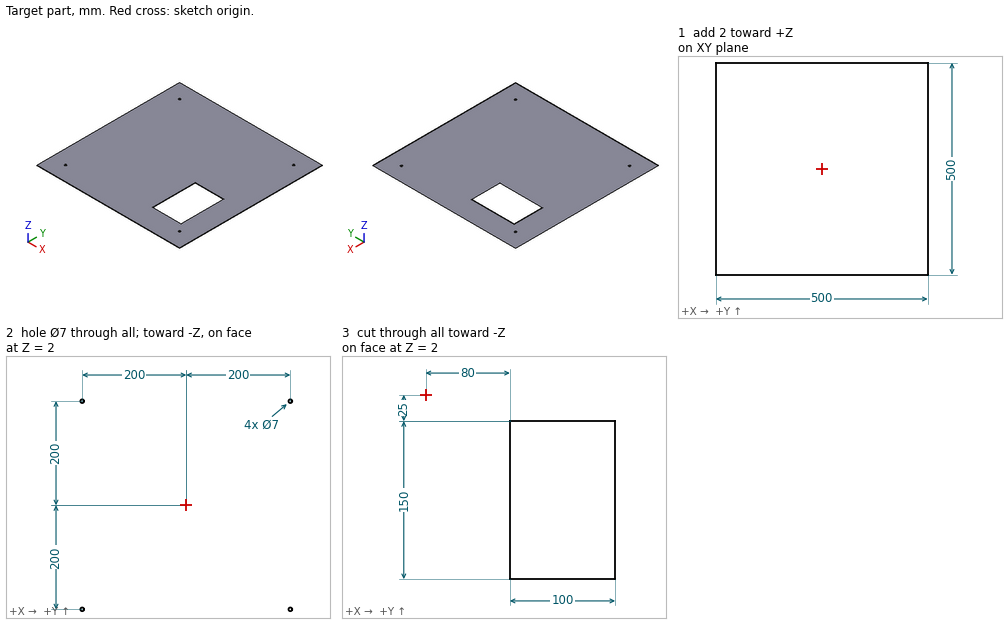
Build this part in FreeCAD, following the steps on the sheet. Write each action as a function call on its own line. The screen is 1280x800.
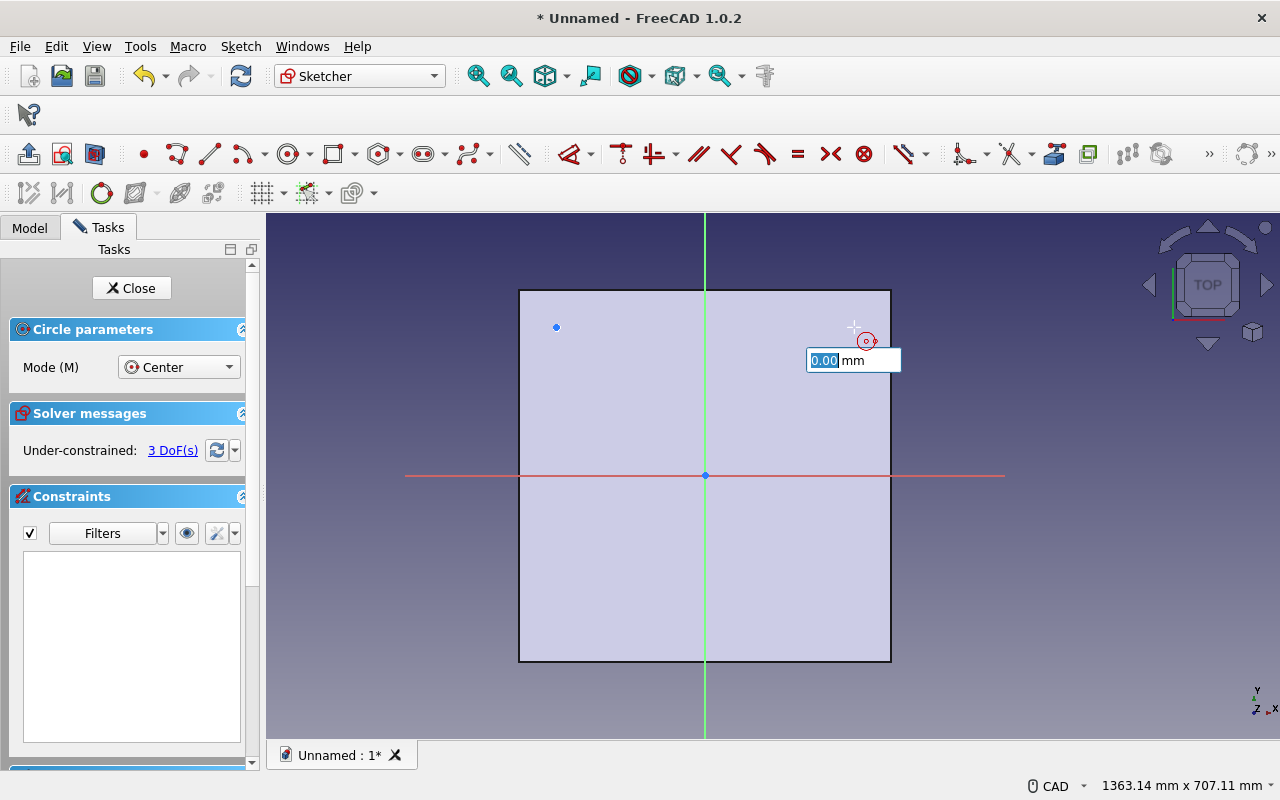
scroll(856, 325, up, 10)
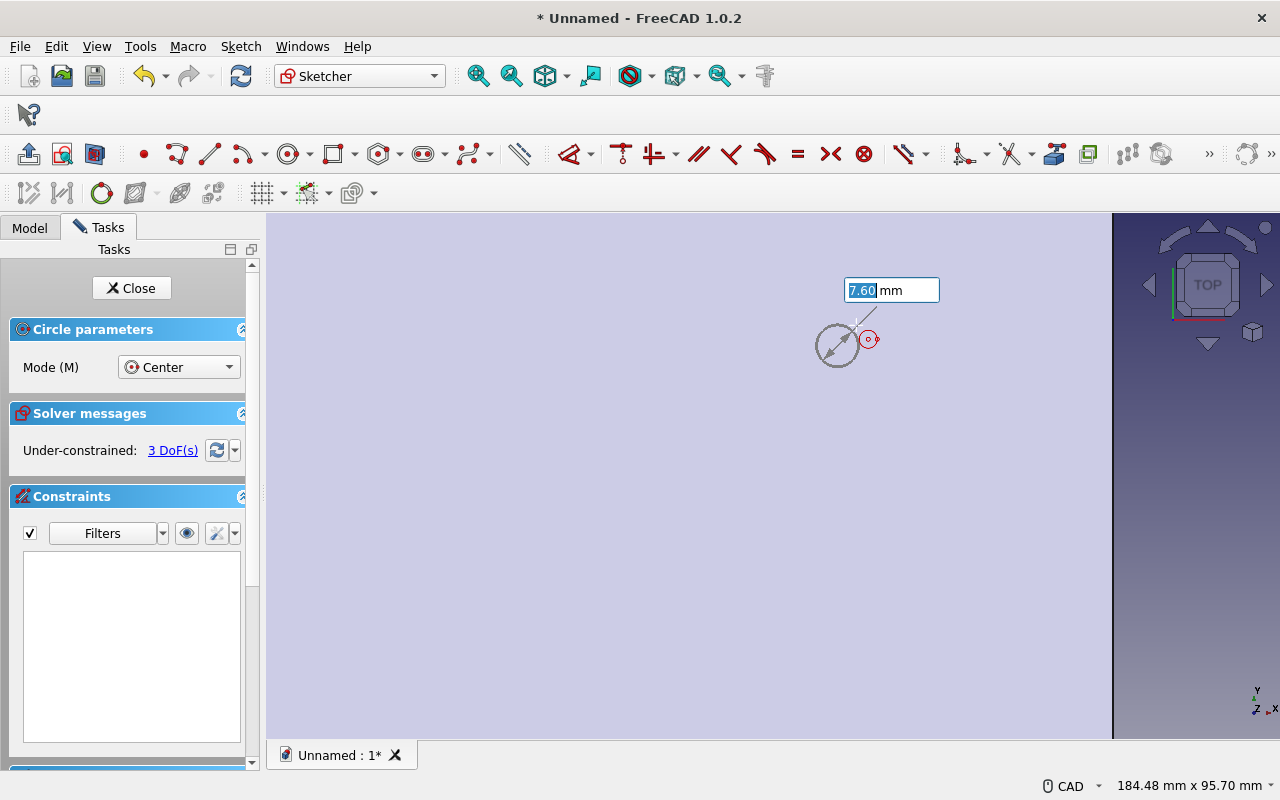
click(852, 326)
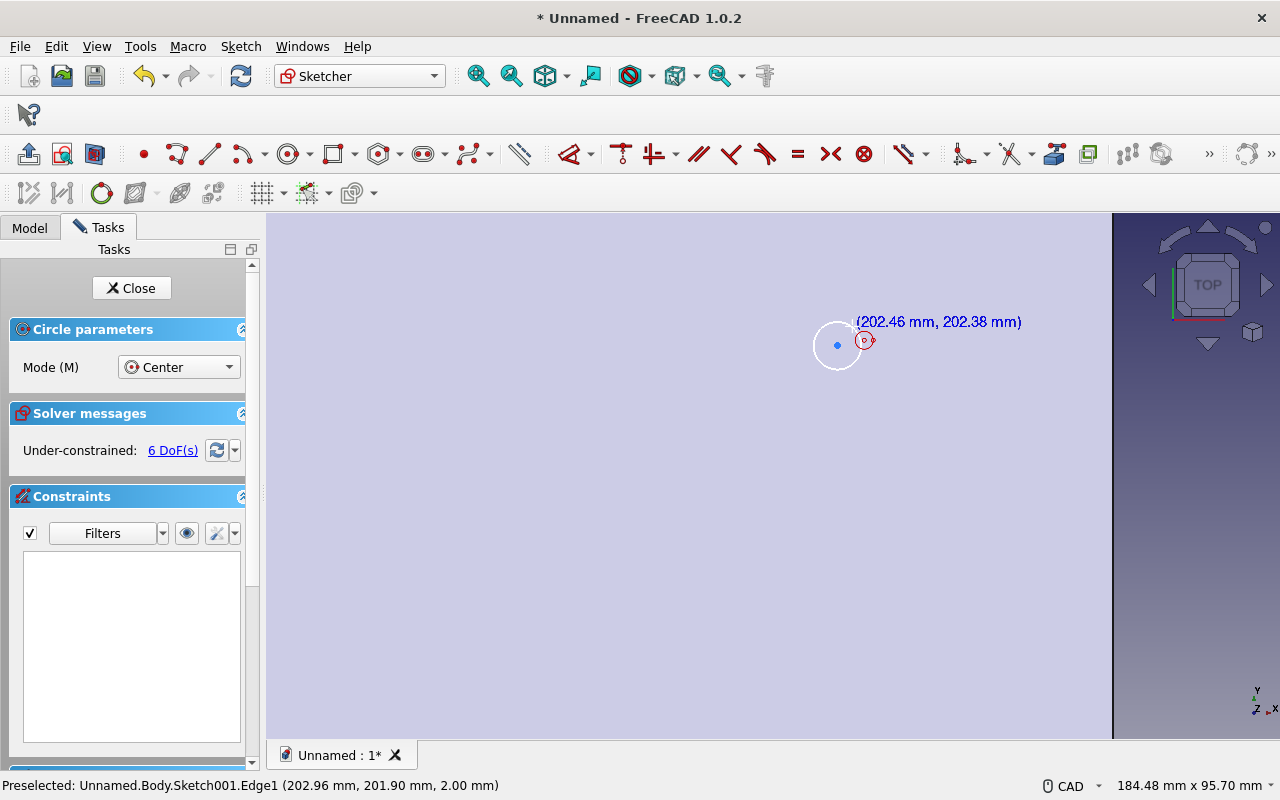
scroll(856, 325, down, 10)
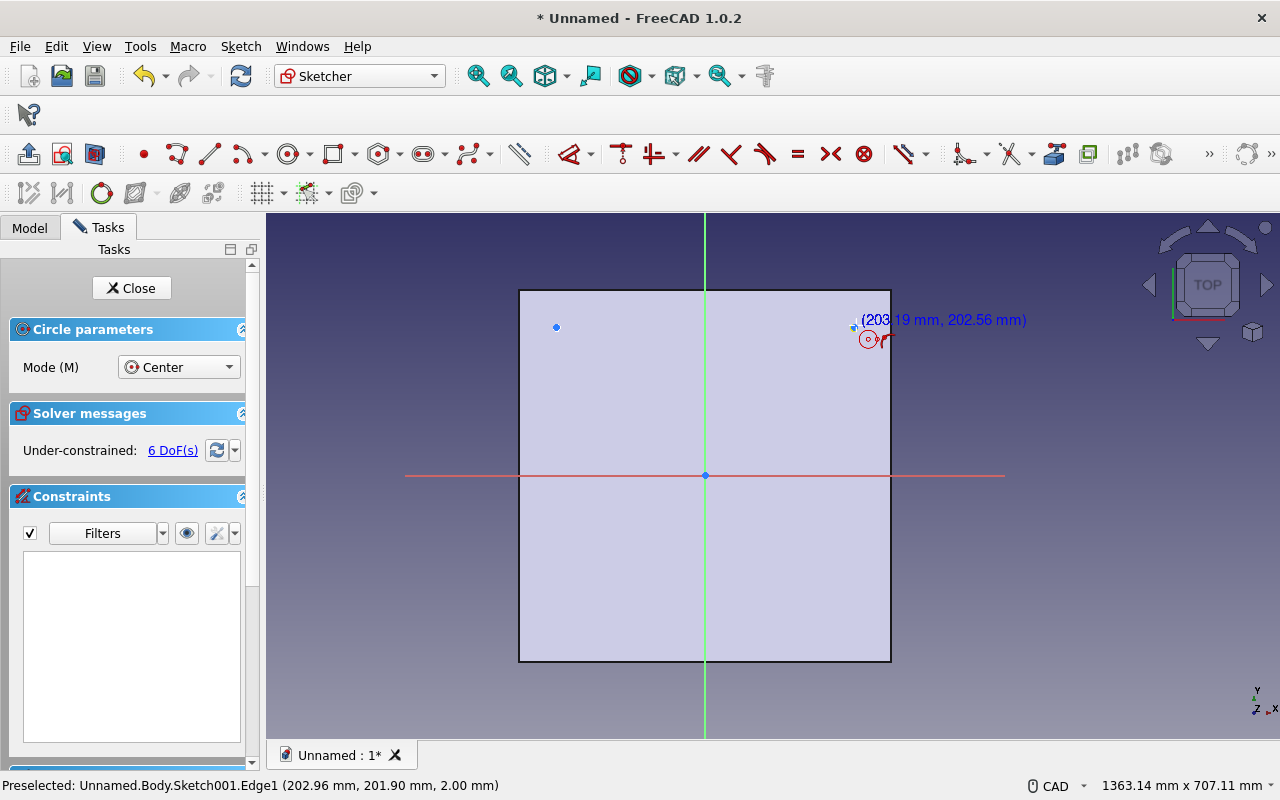
scroll(557, 625, up, 11)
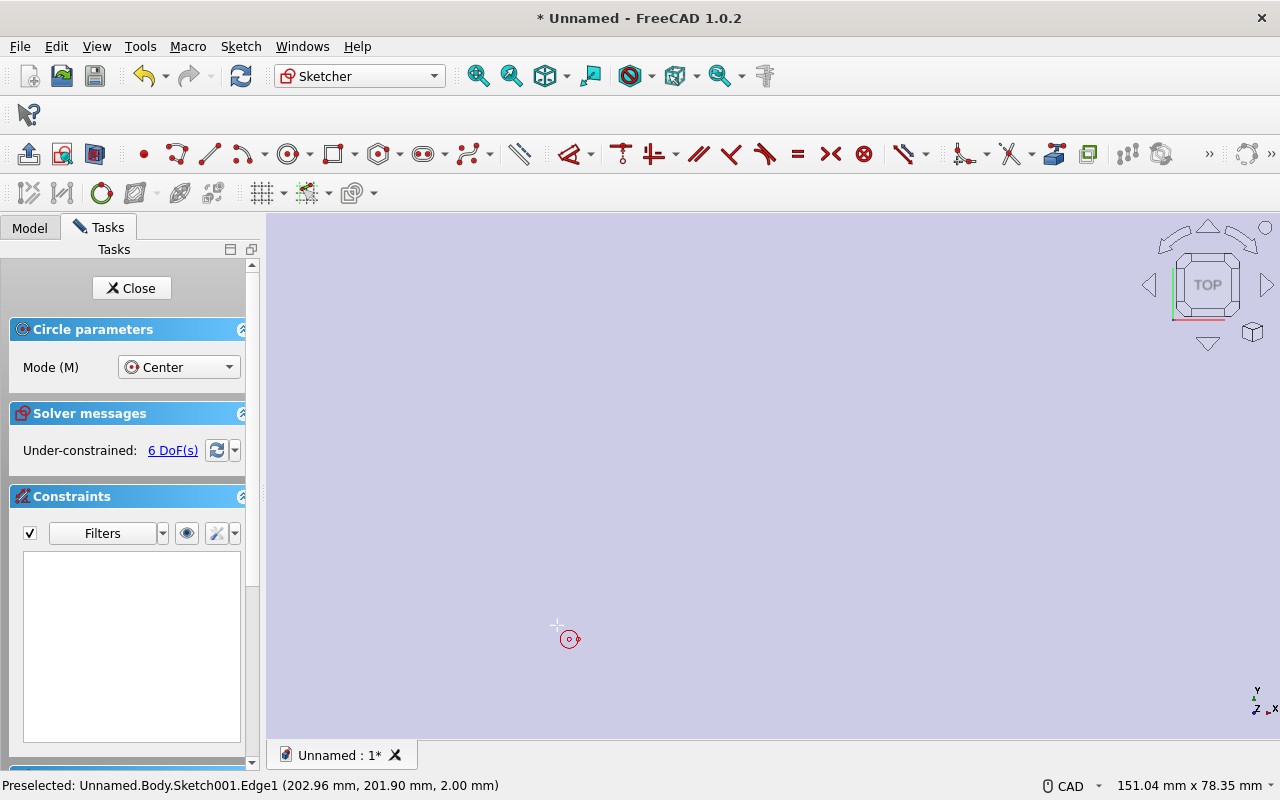
scroll(556, 626, down, 11)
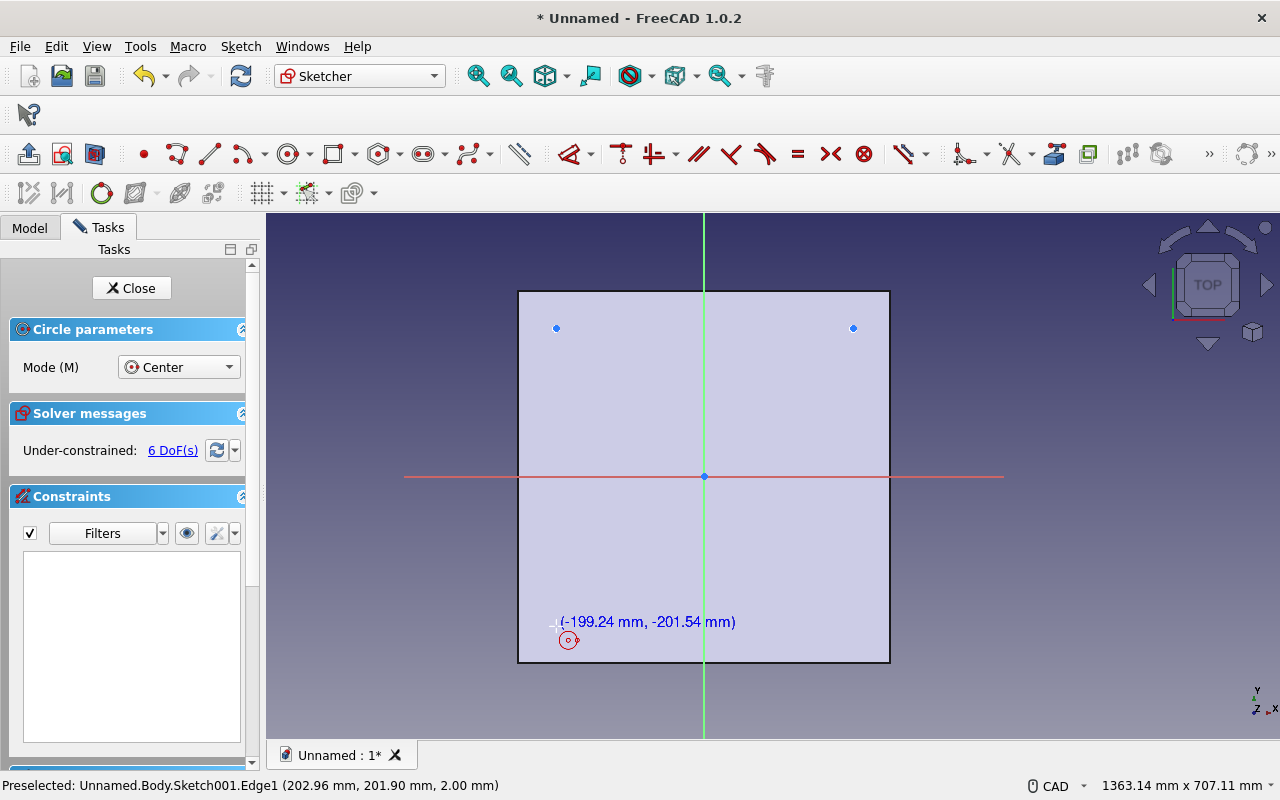
click(556, 626)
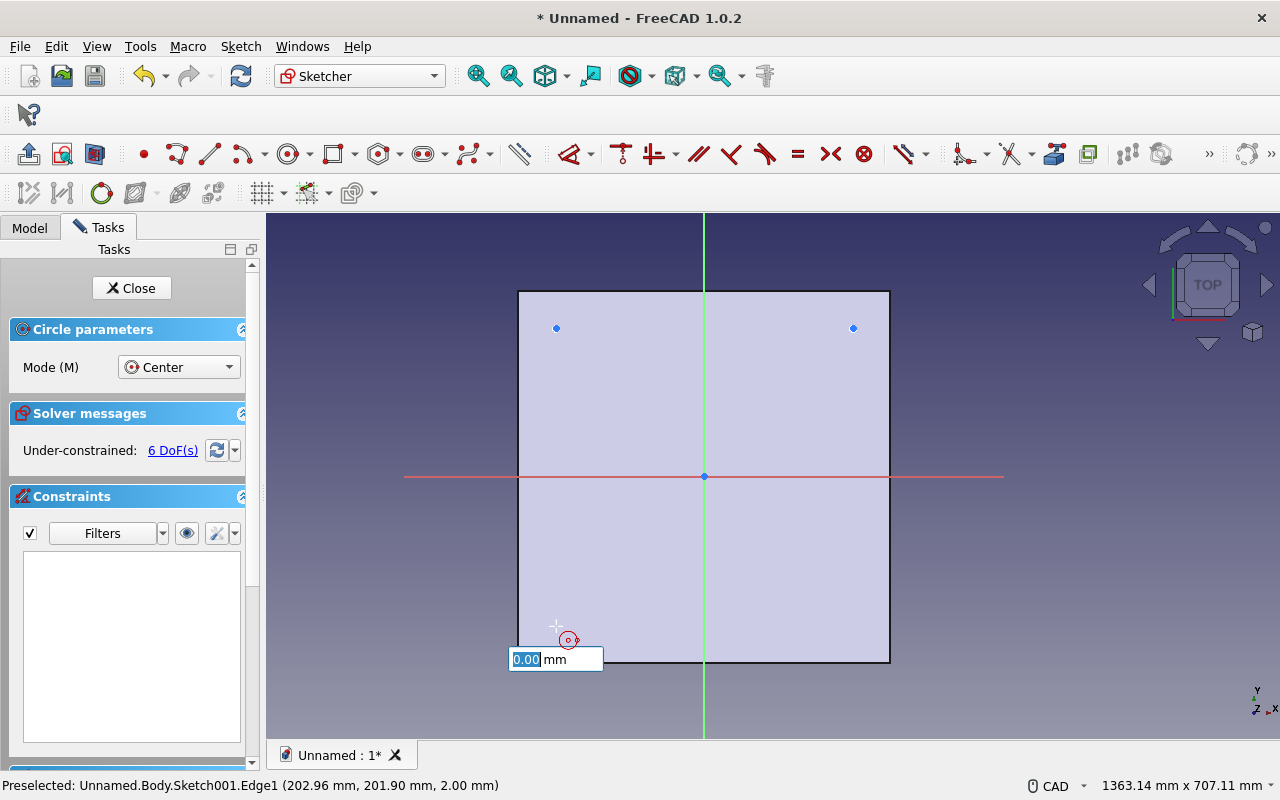
scroll(558, 624, up, 10)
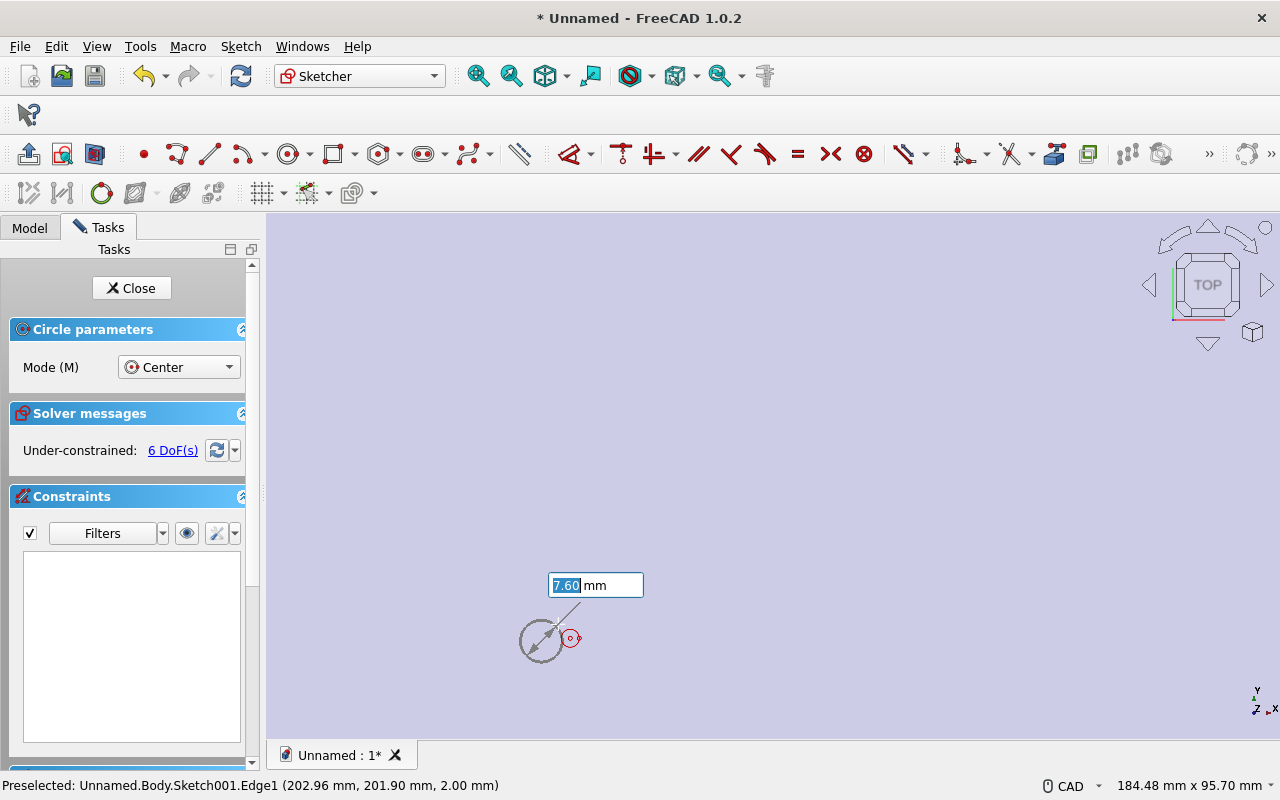
click(553, 618)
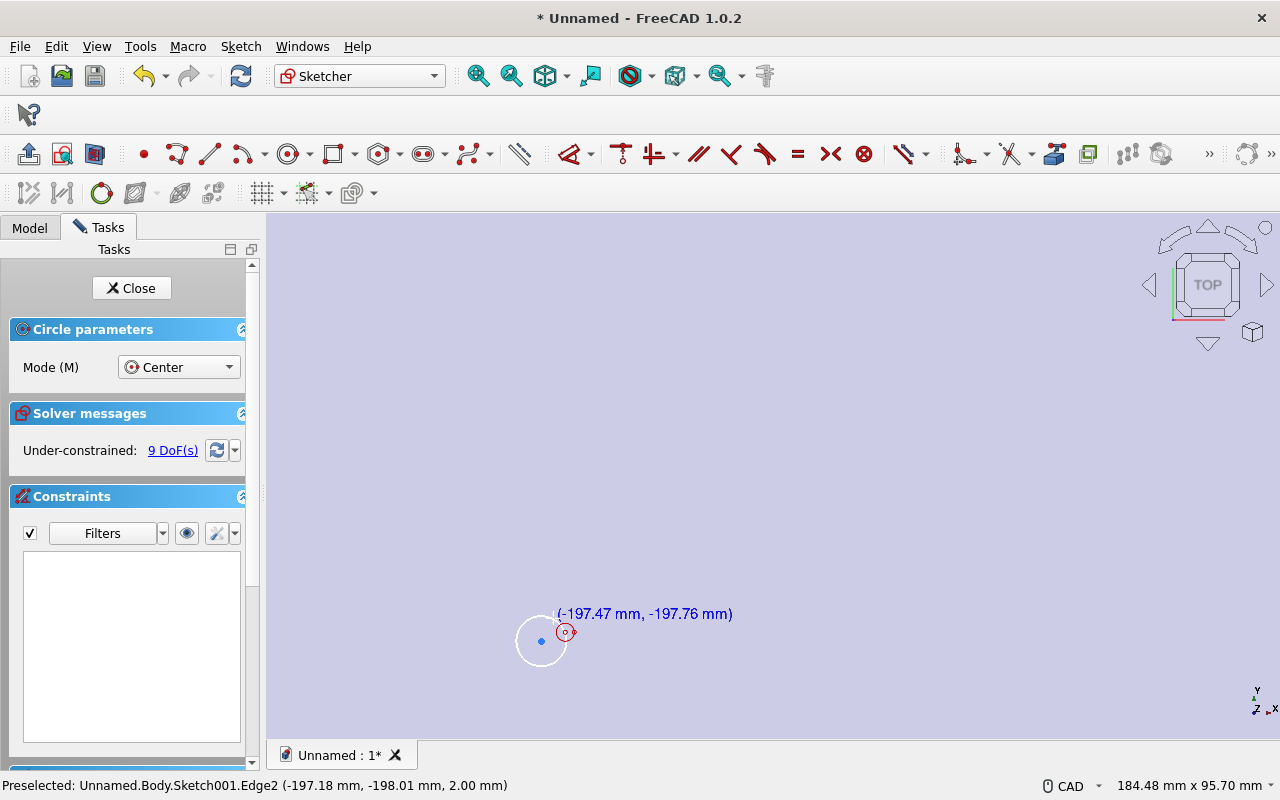
scroll(558, 624, down, 10)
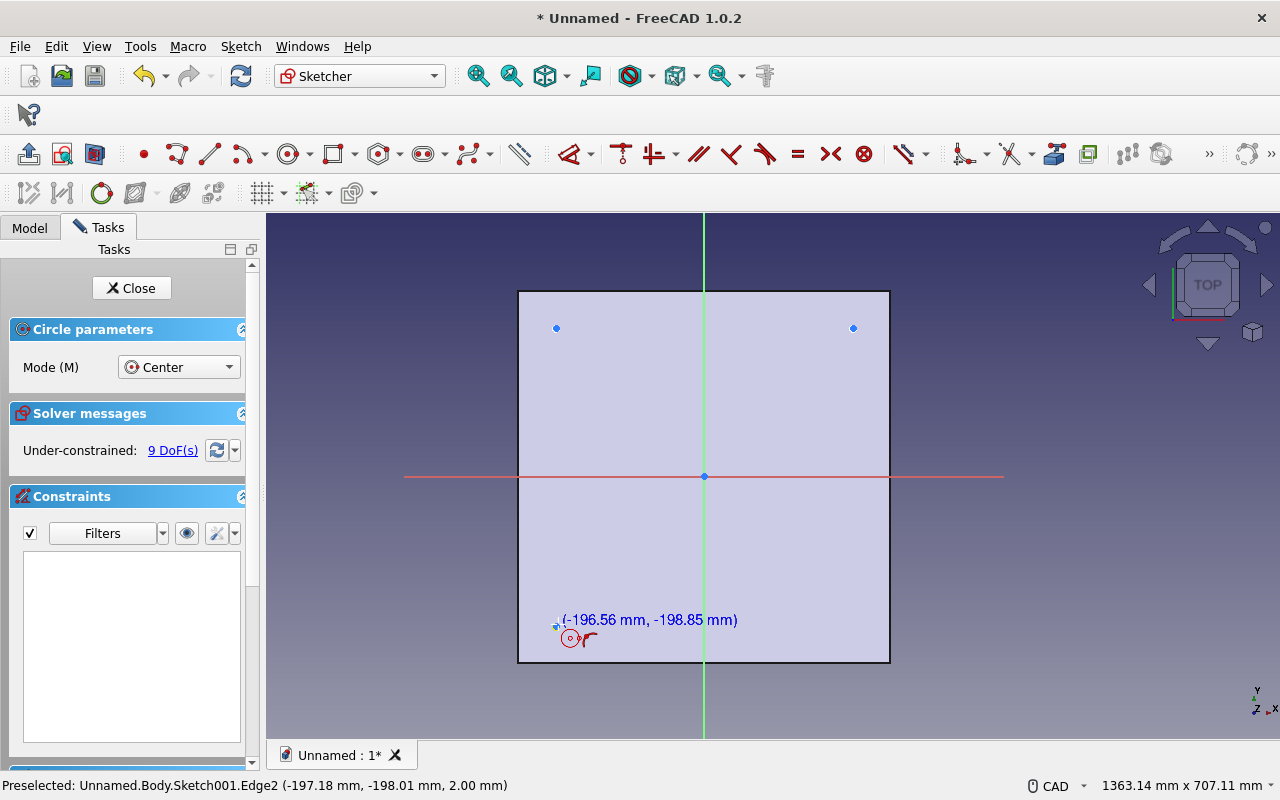
scroll(853, 626, up, 11)